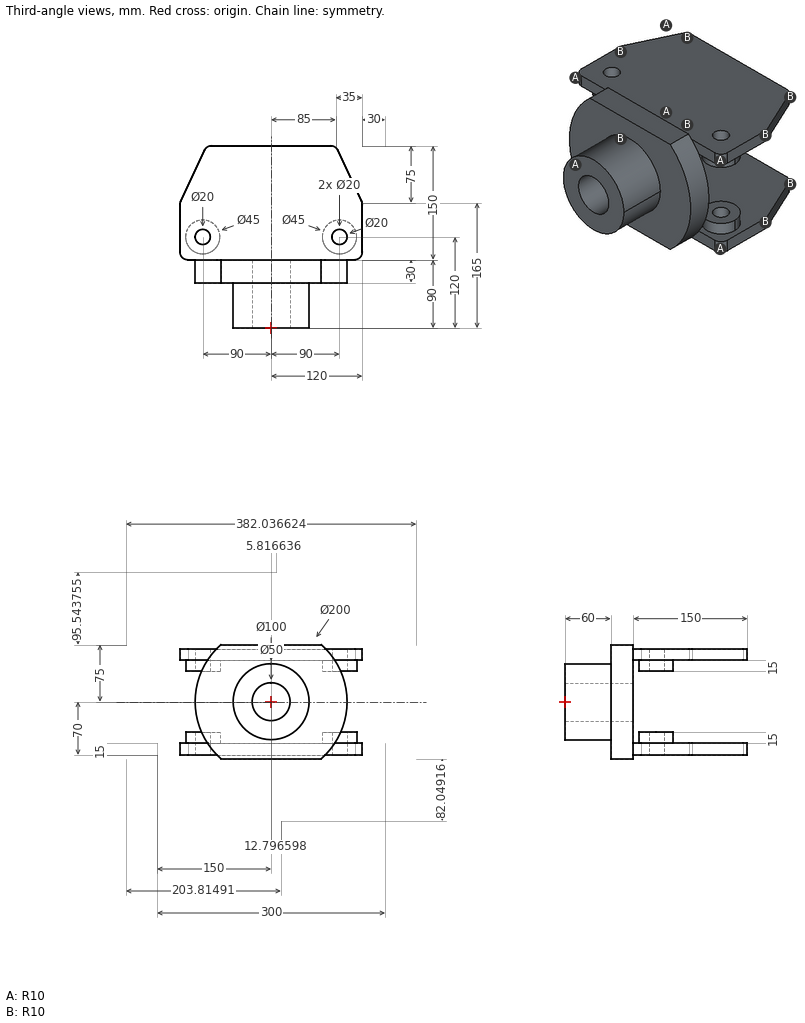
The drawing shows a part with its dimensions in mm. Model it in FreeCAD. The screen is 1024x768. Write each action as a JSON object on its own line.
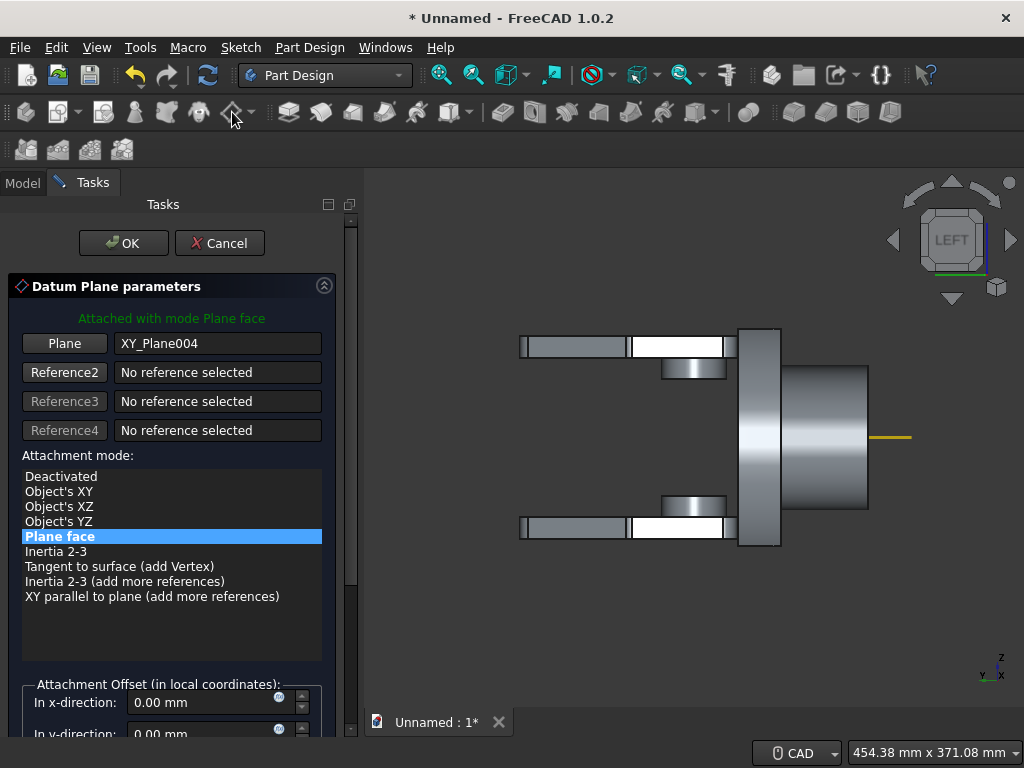
{"action": "scroll", "coordinate": [351, 475], "scroll_direction": "down", "scroll_amount": 2}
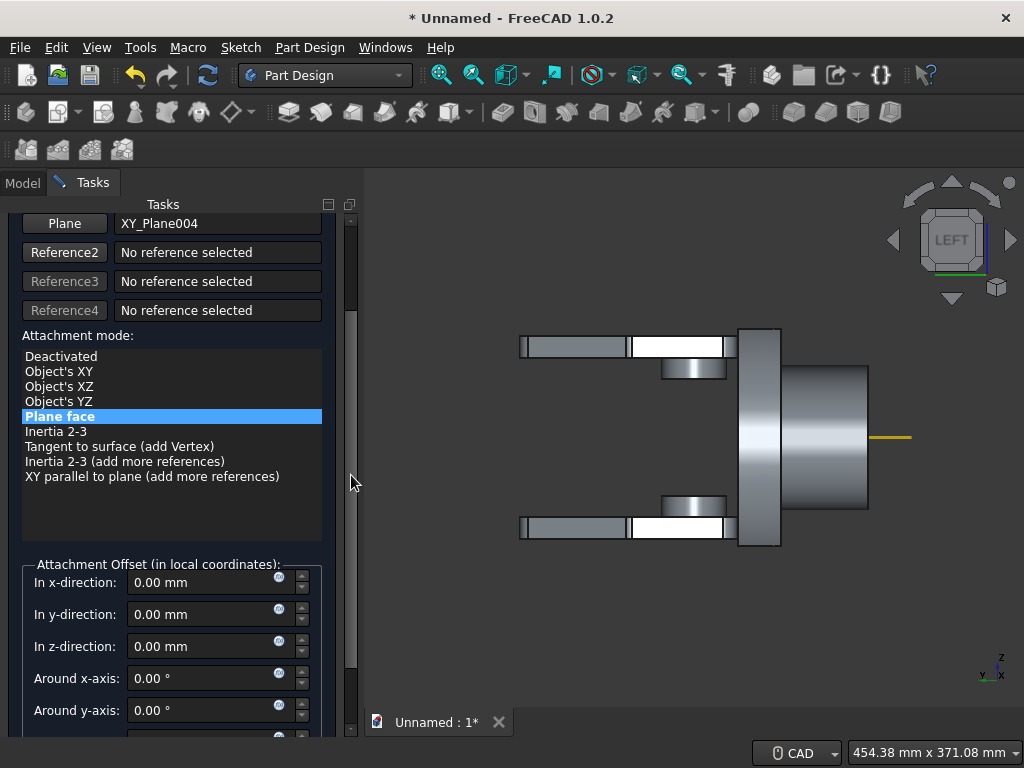
{"action": "triple_click", "coordinate": [210, 646]}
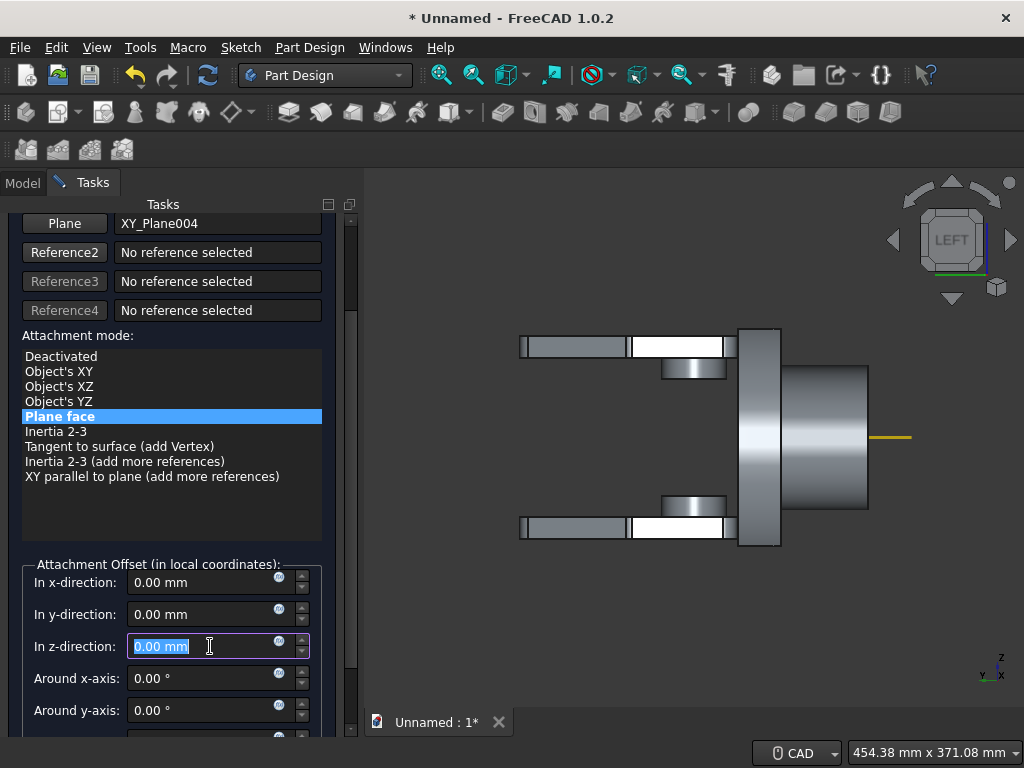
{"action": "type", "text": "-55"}
{"action": "key", "text": "Tab"}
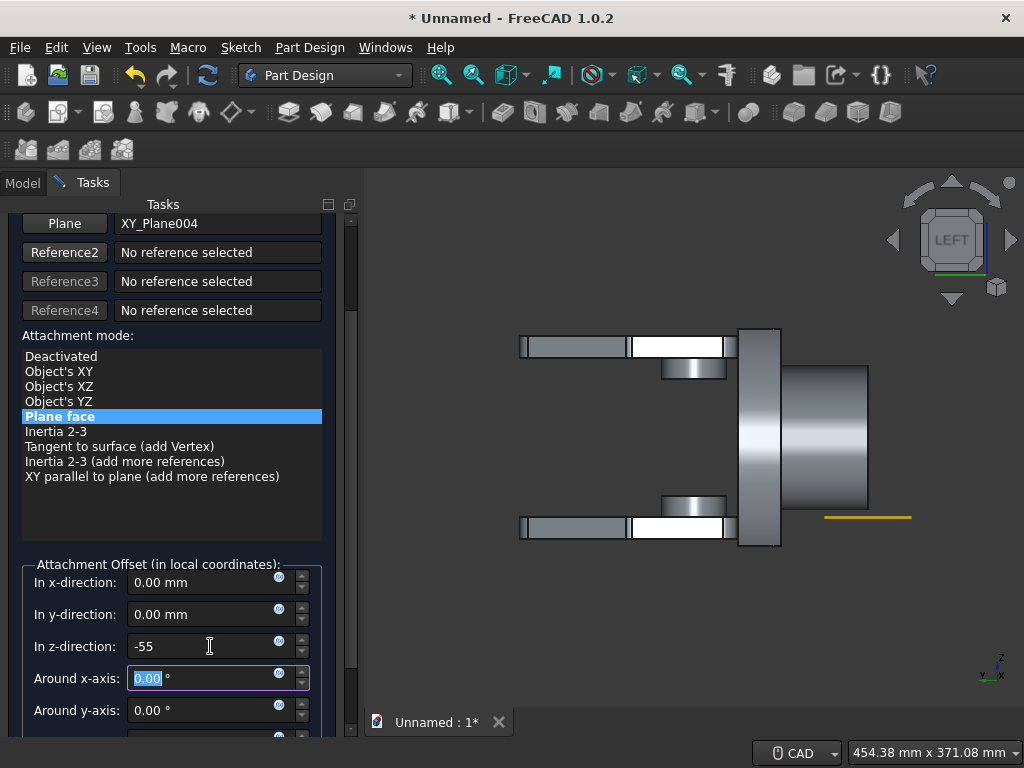
{"action": "scroll", "coordinate": [351, 475], "scroll_direction": "up", "scroll_amount": 3}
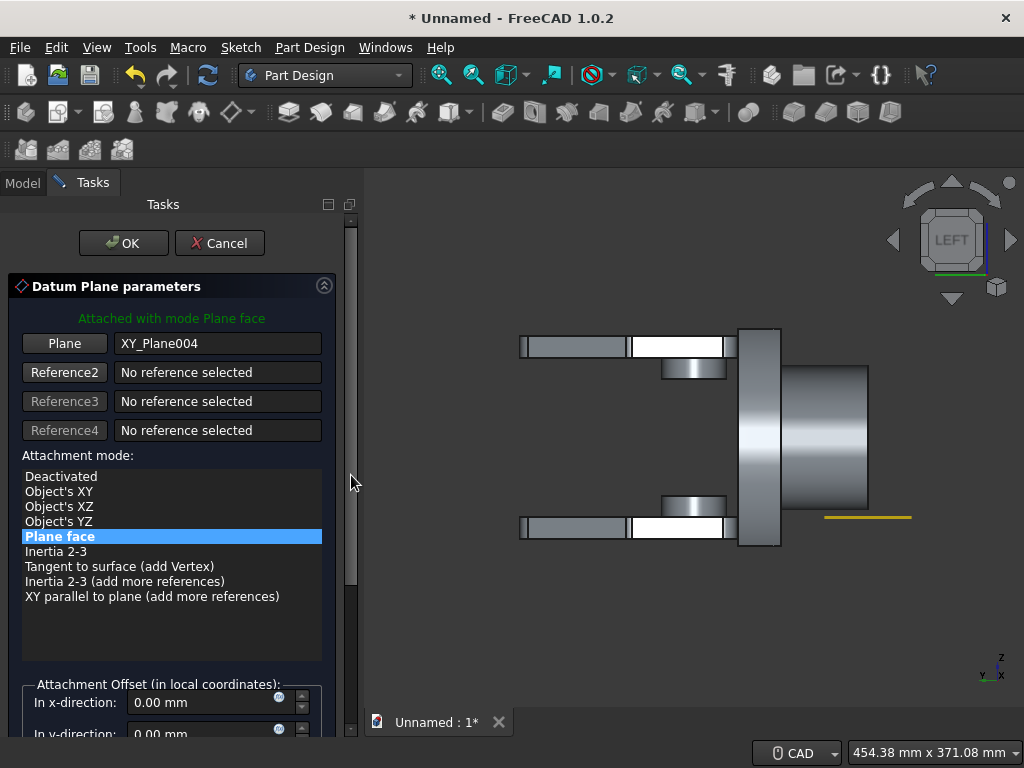
{"action": "left_click", "coordinate": [124, 243]}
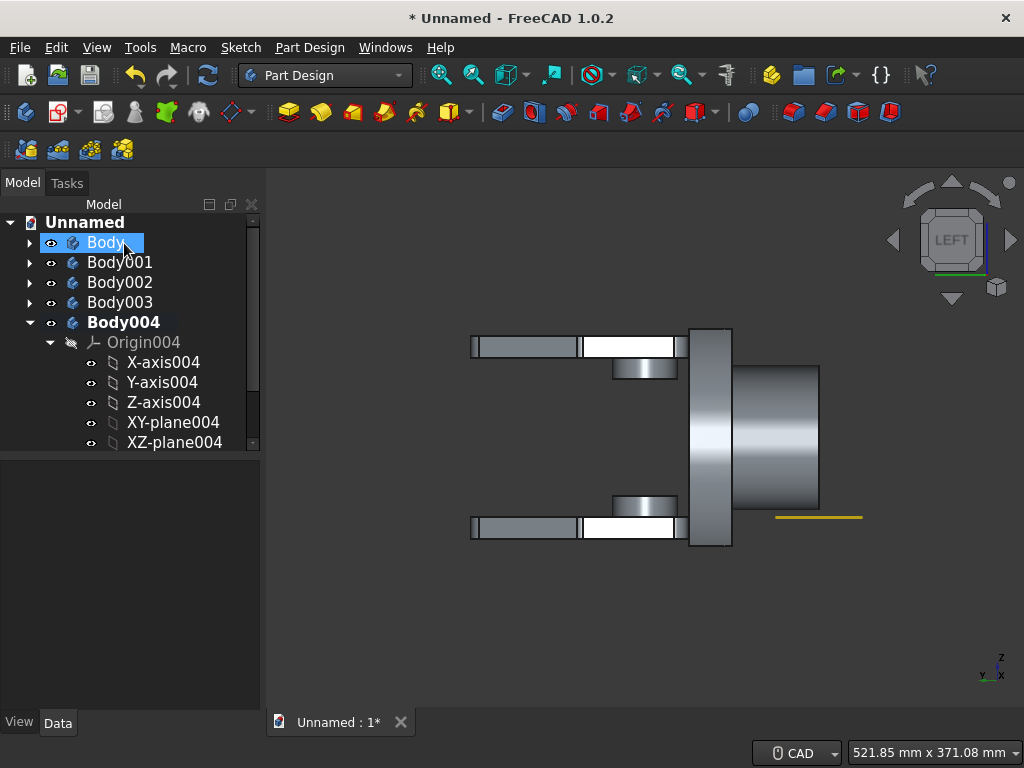
{"action": "scroll", "coordinate": [100, 338], "scroll_direction": "down", "scroll_amount": 3}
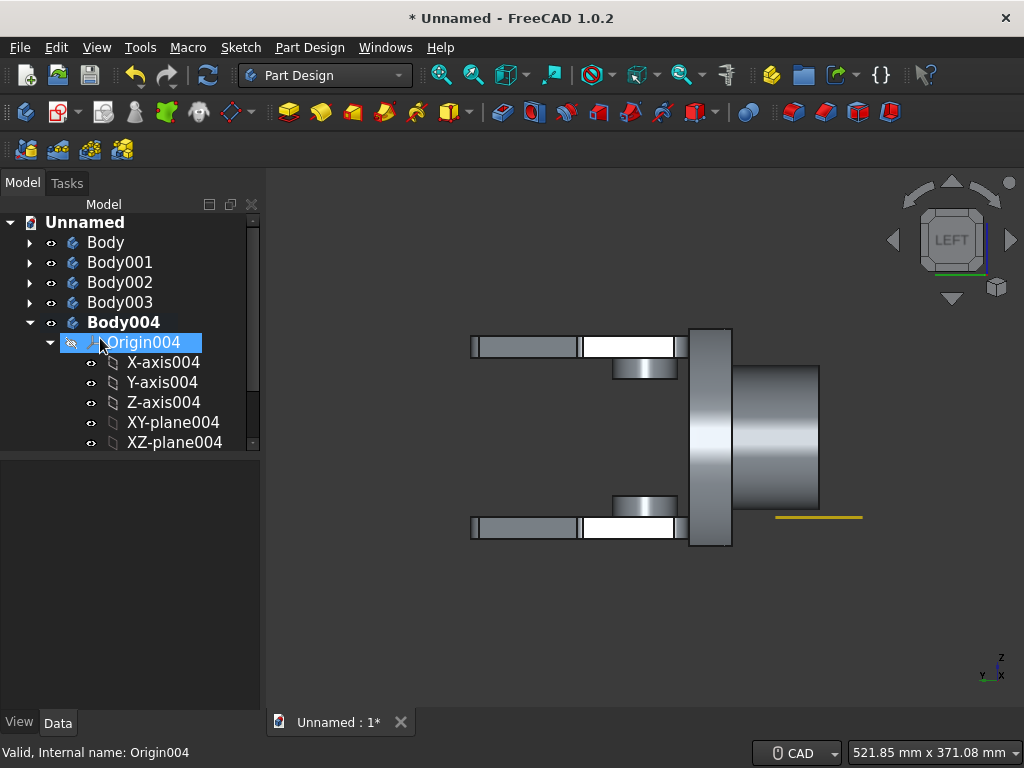
{"action": "left_click", "coordinate": [116, 423]}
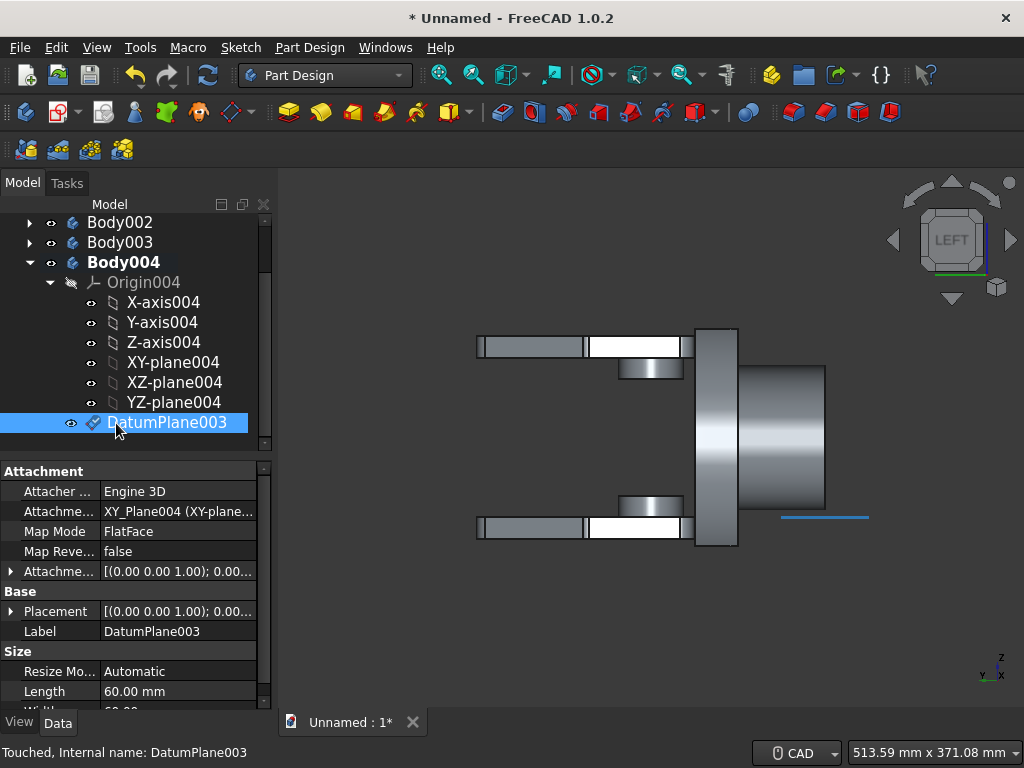
{"action": "left_click", "coordinate": [58, 112]}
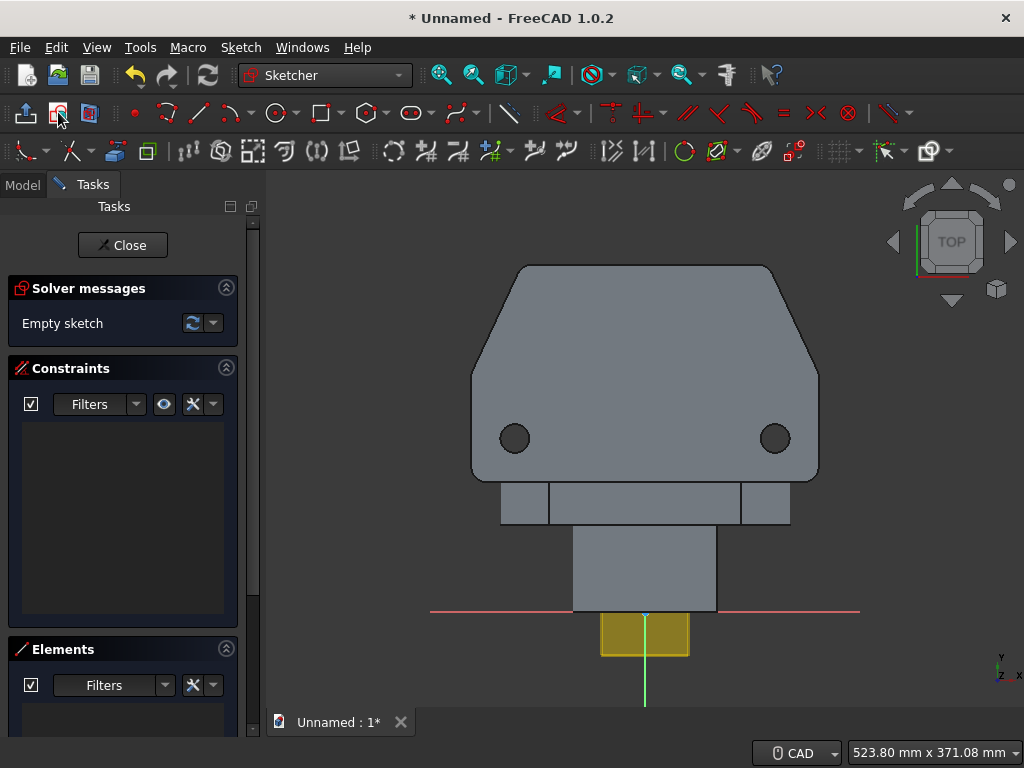
{"action": "scroll", "coordinate": [499, 439], "scroll_direction": "up", "scroll_amount": 8}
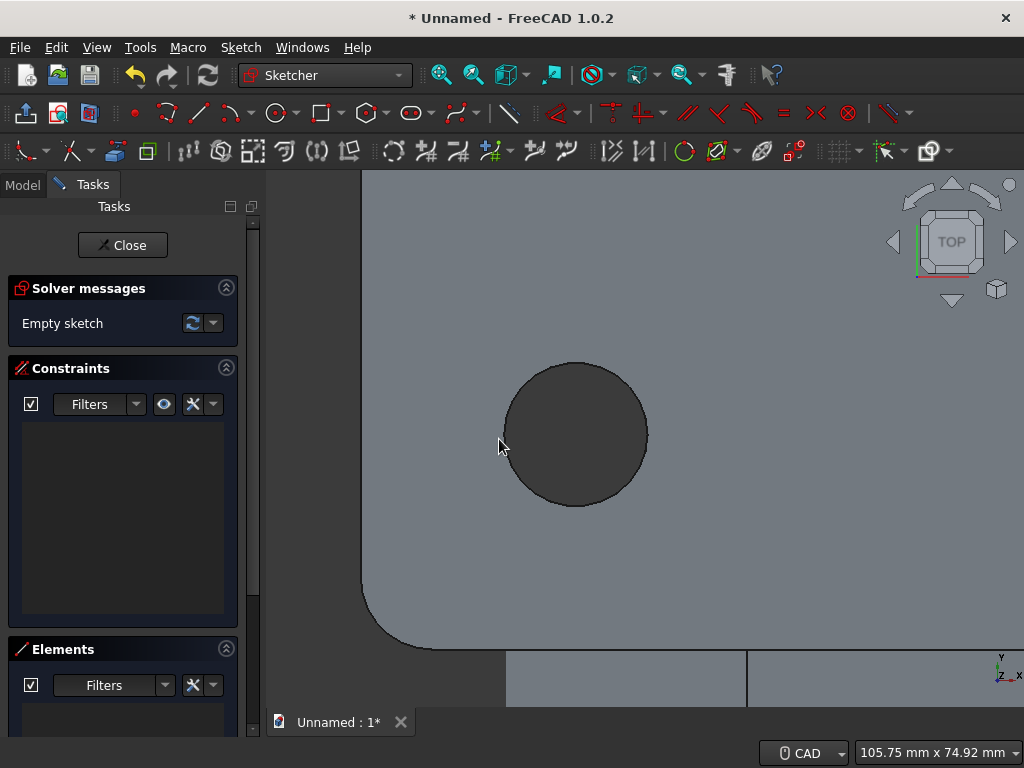
{"action": "left_click", "coordinate": [276, 114]}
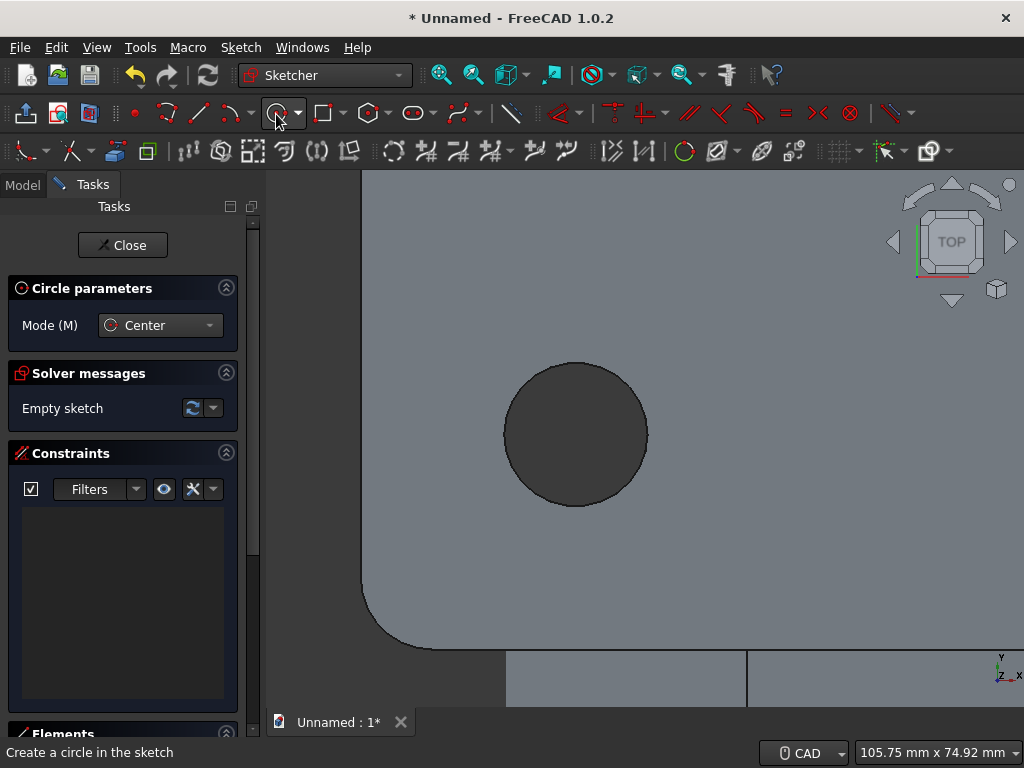
{"action": "left_click", "coordinate": [576, 435]}
{"action": "left_click", "coordinate": [690, 321]}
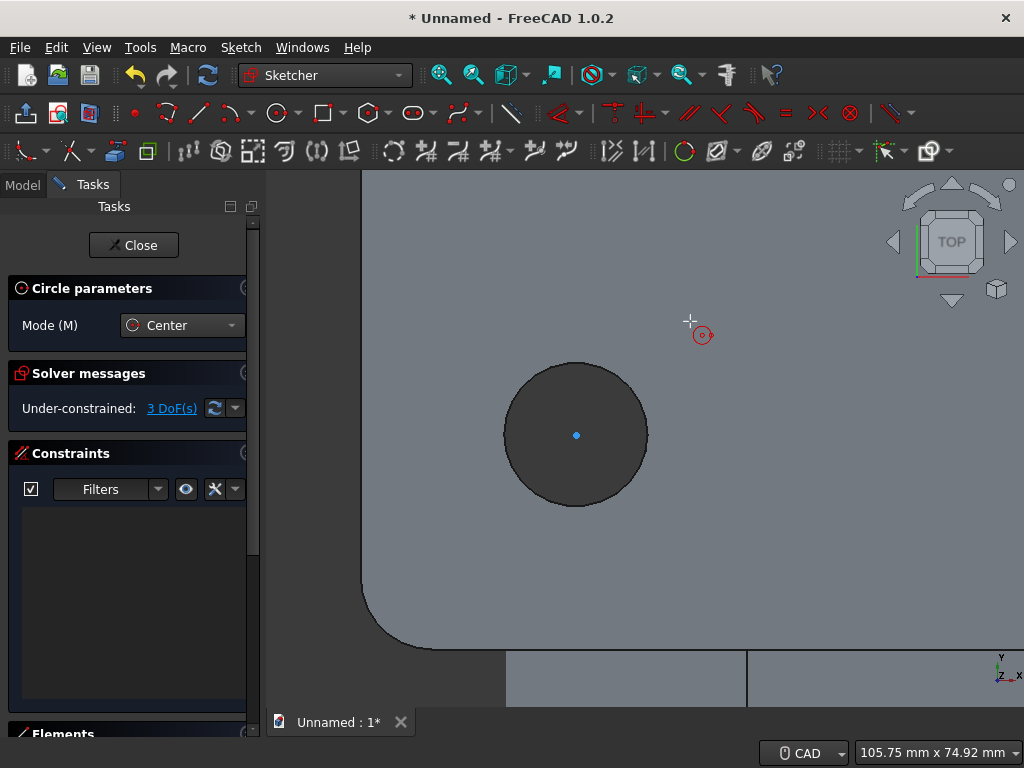
{"action": "left_click", "coordinate": [576, 436]}
{"action": "left_click", "coordinate": [627, 384]}
{"action": "key", "text": "Escape"}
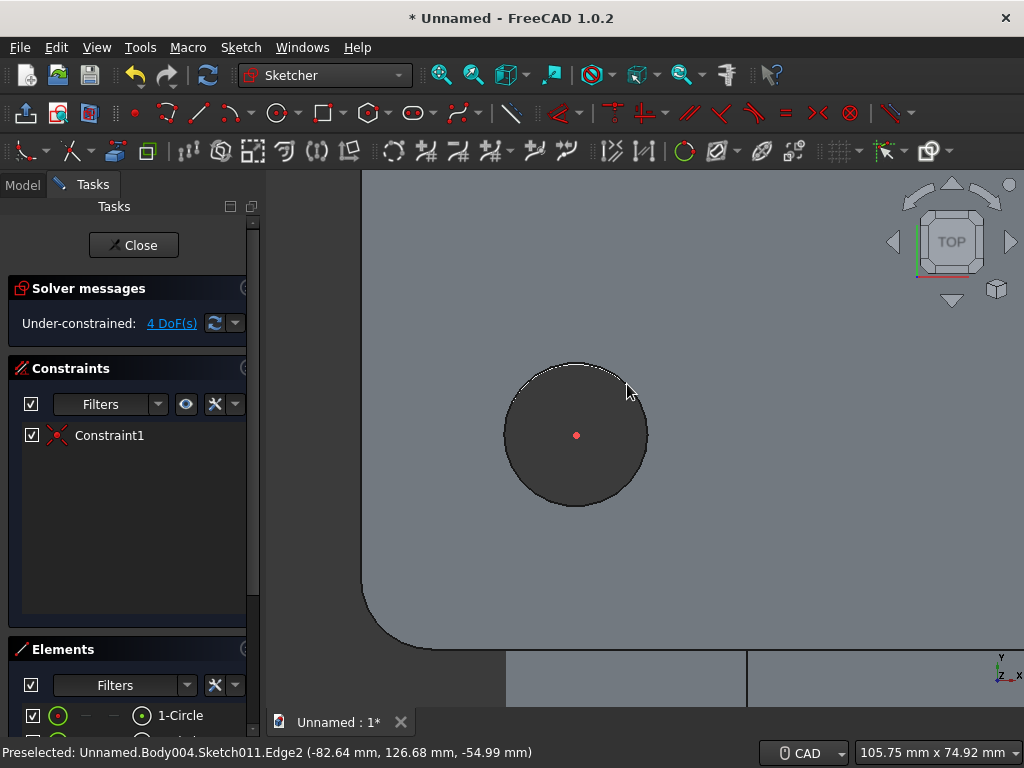
{"action": "left_click", "coordinate": [558, 114]}